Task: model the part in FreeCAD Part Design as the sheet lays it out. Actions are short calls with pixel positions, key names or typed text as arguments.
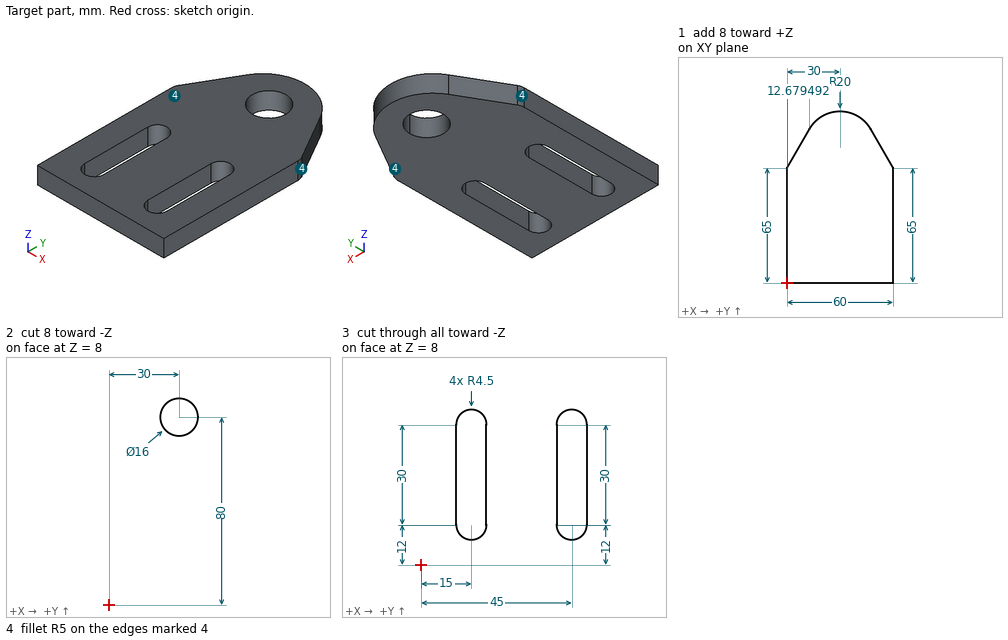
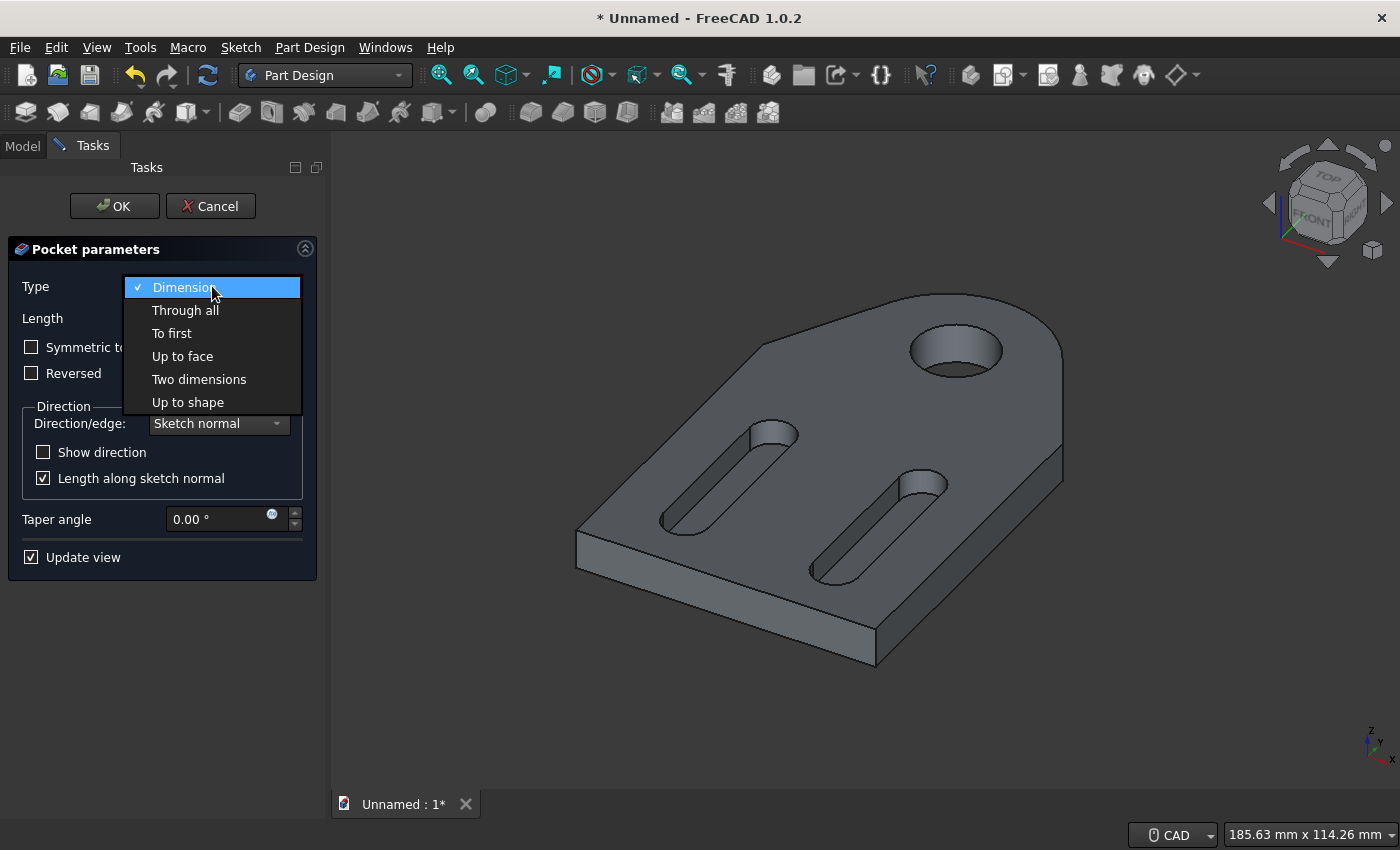
click(212, 310)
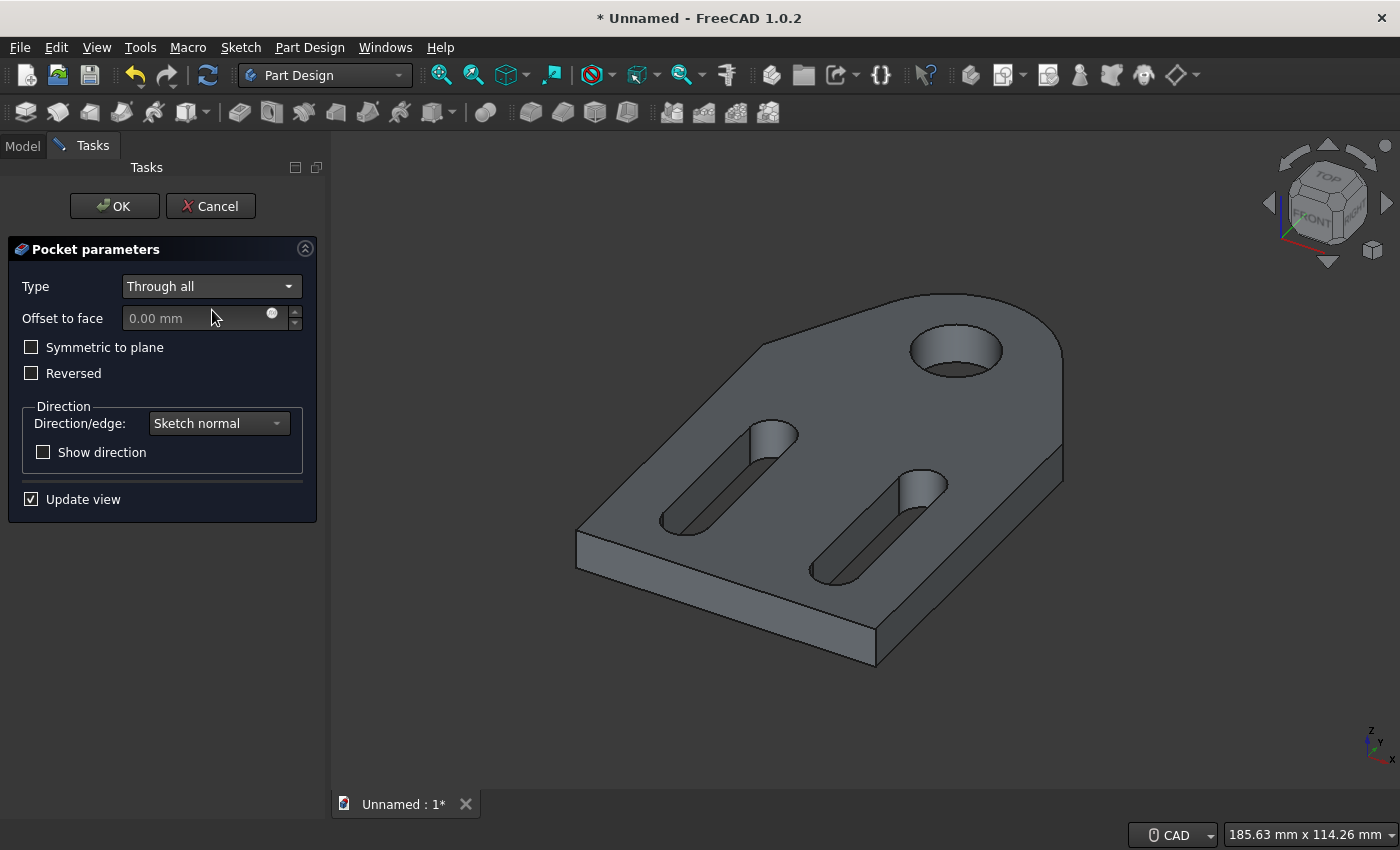
click(115, 206)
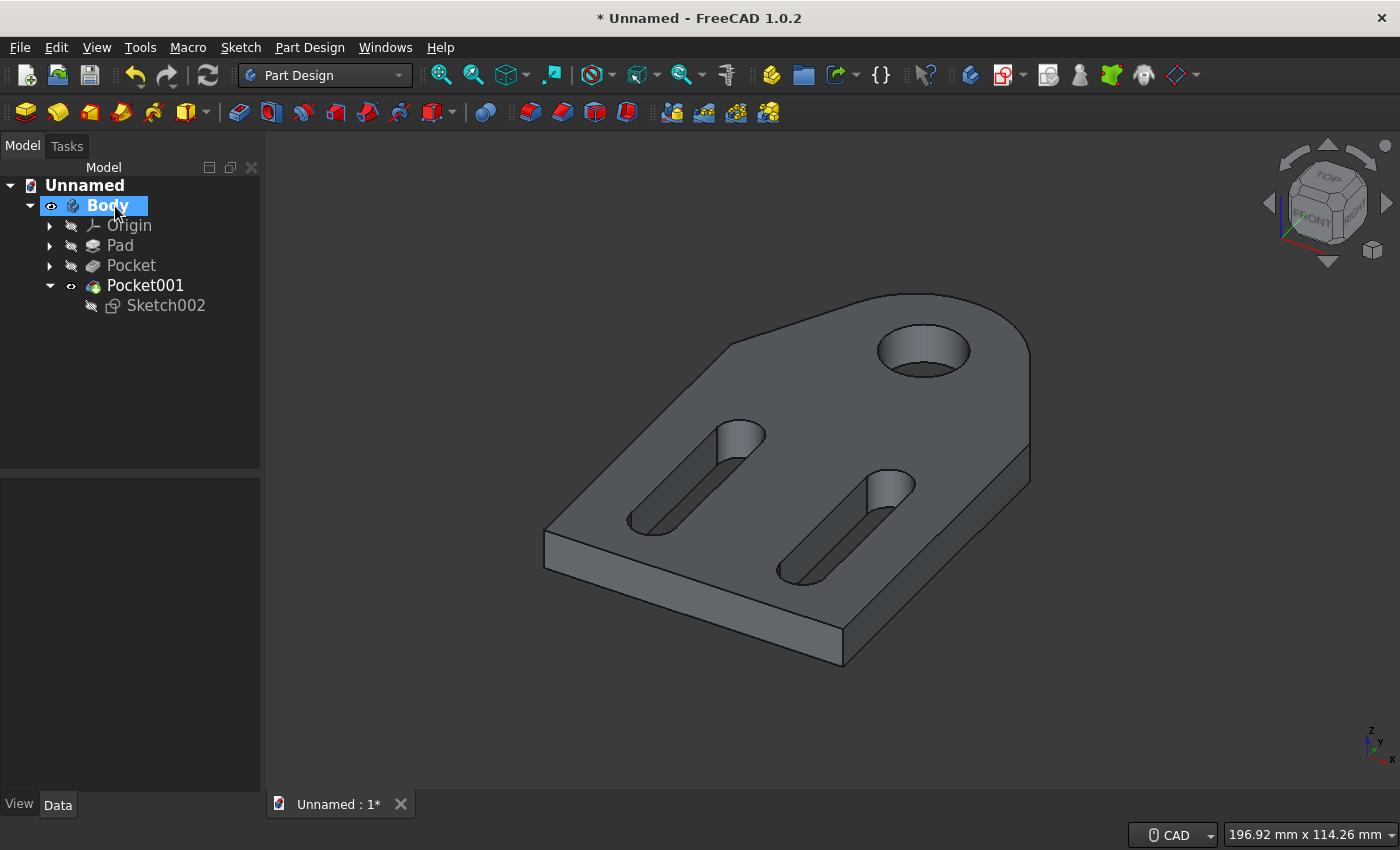
key(0)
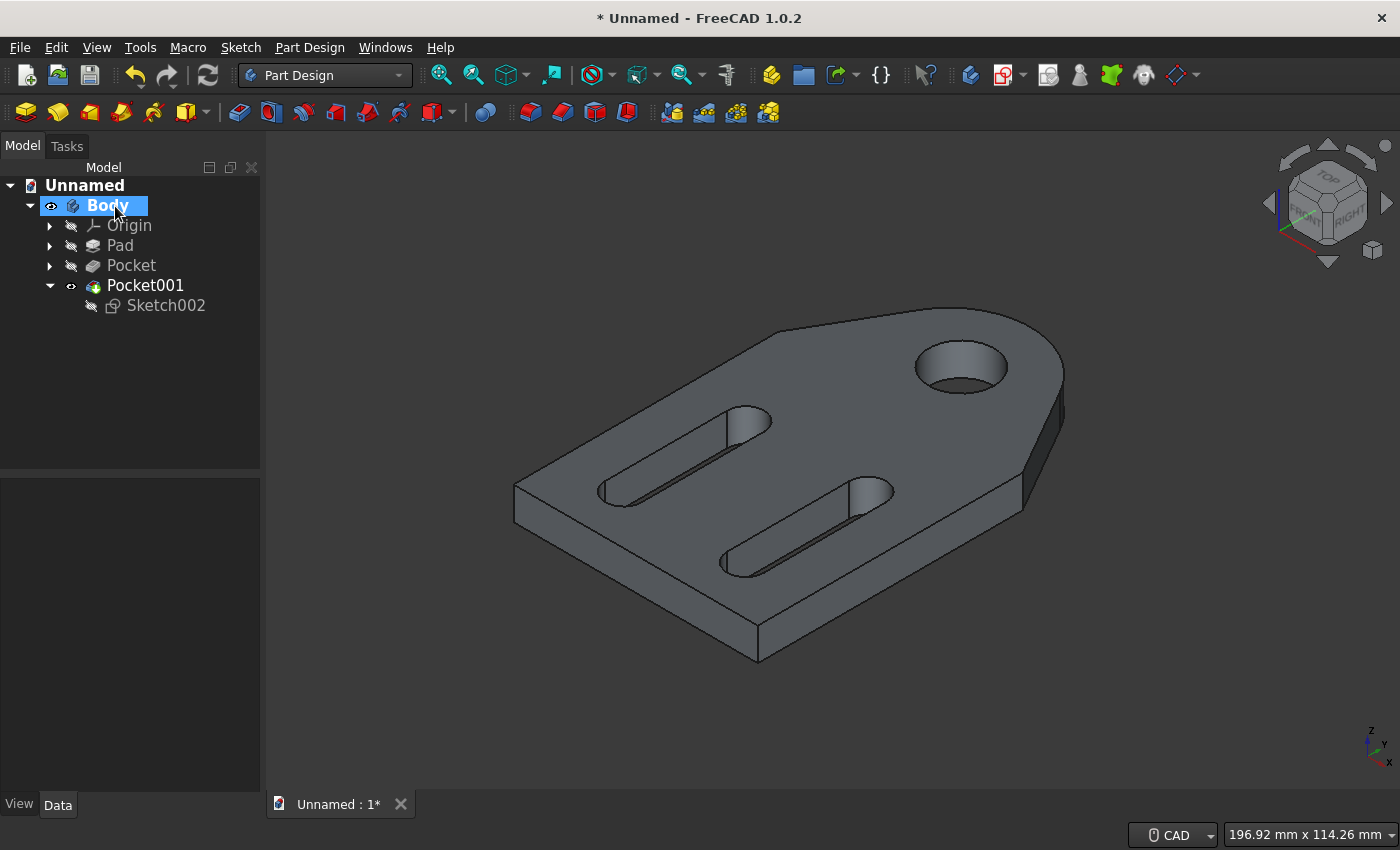
key(2)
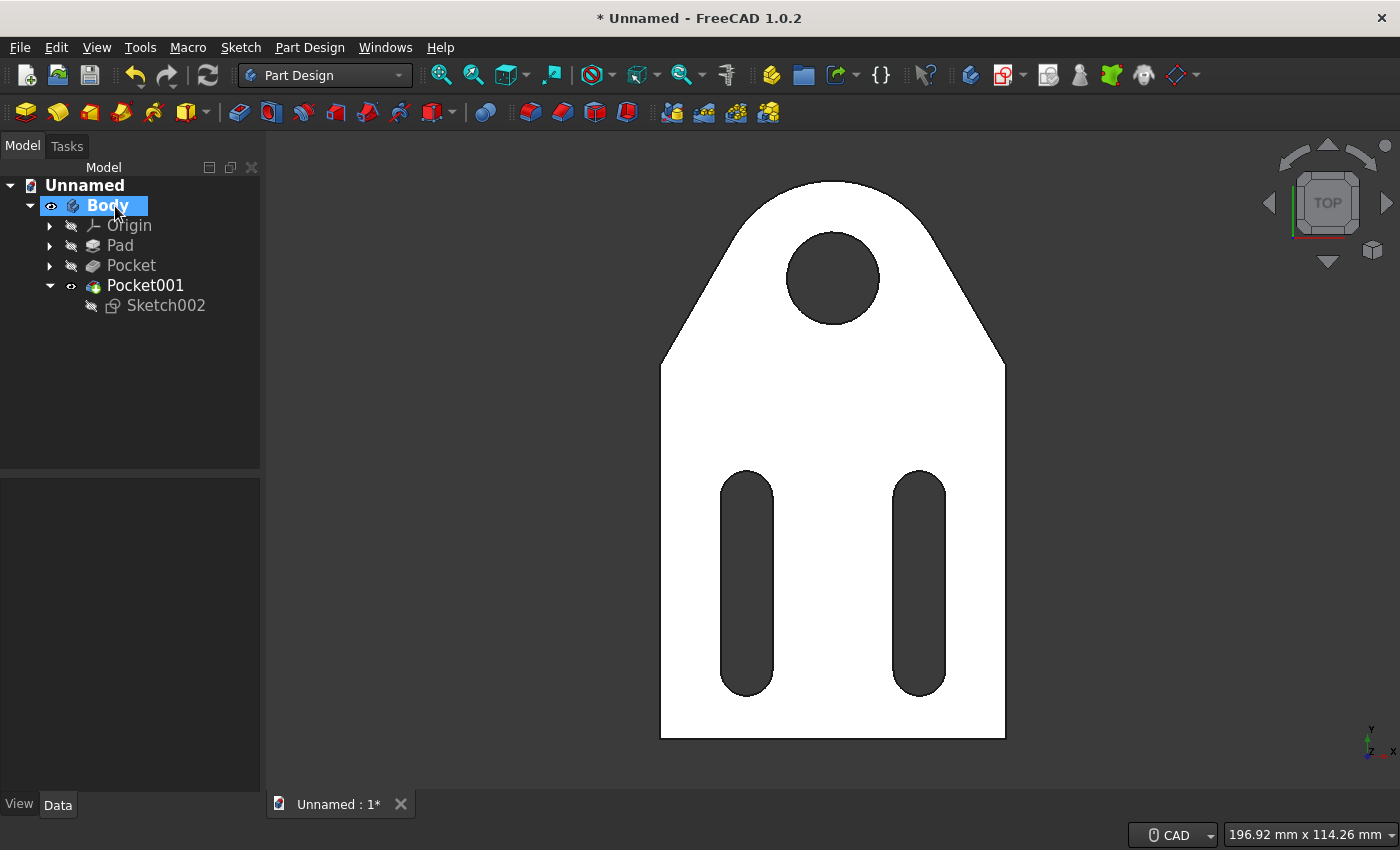
key(1)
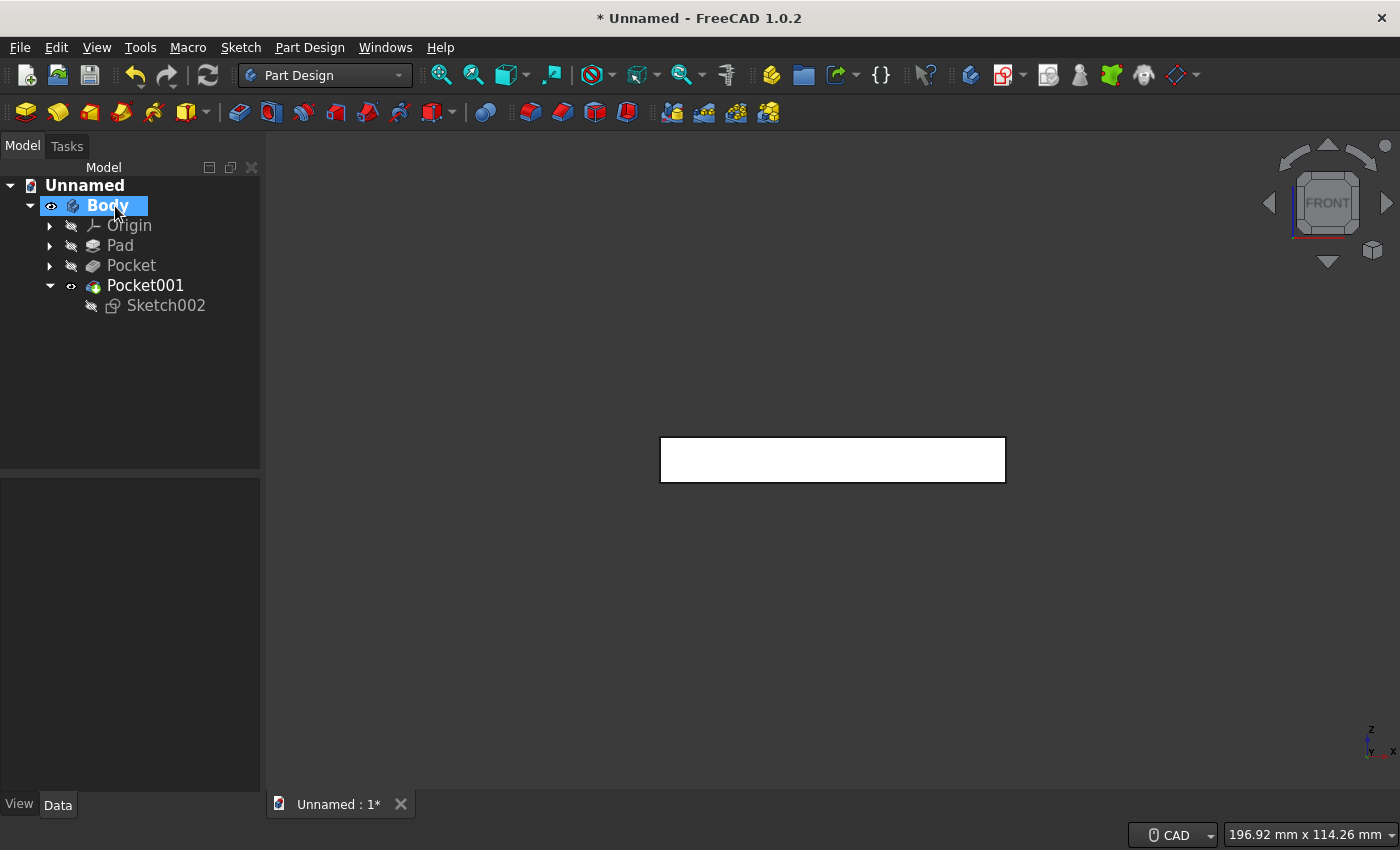
key(v)
key(f)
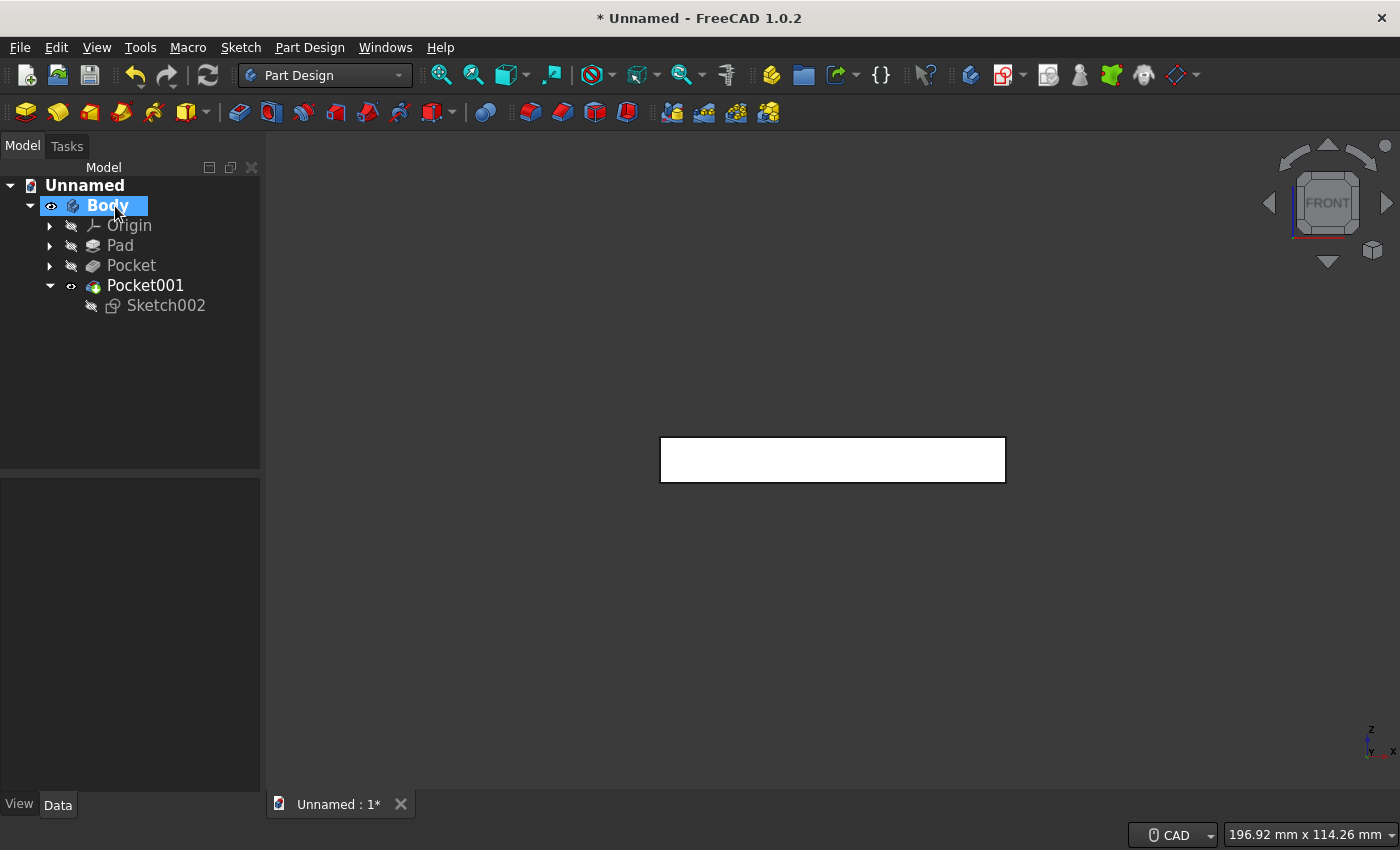
key(3)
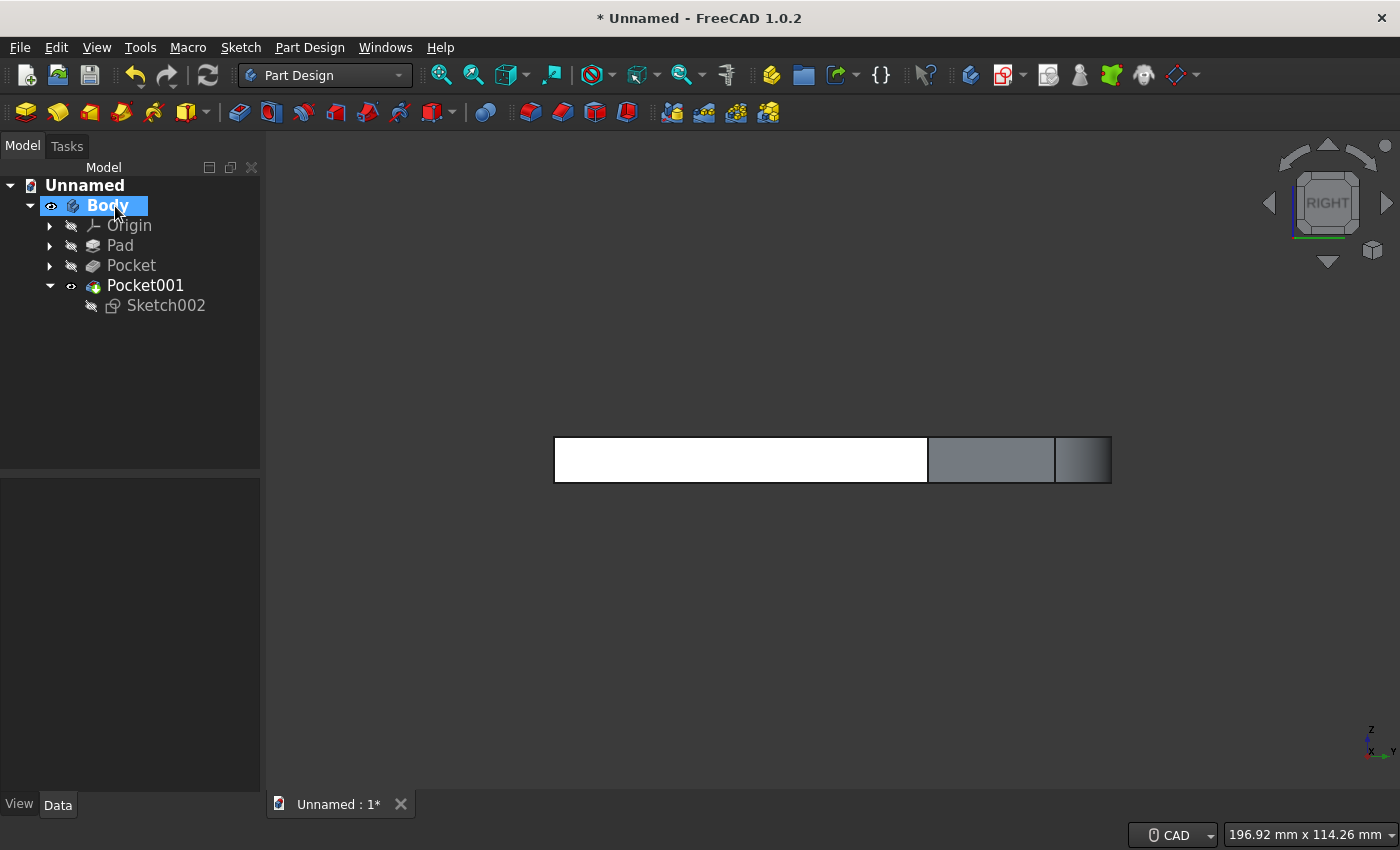
click(928, 459)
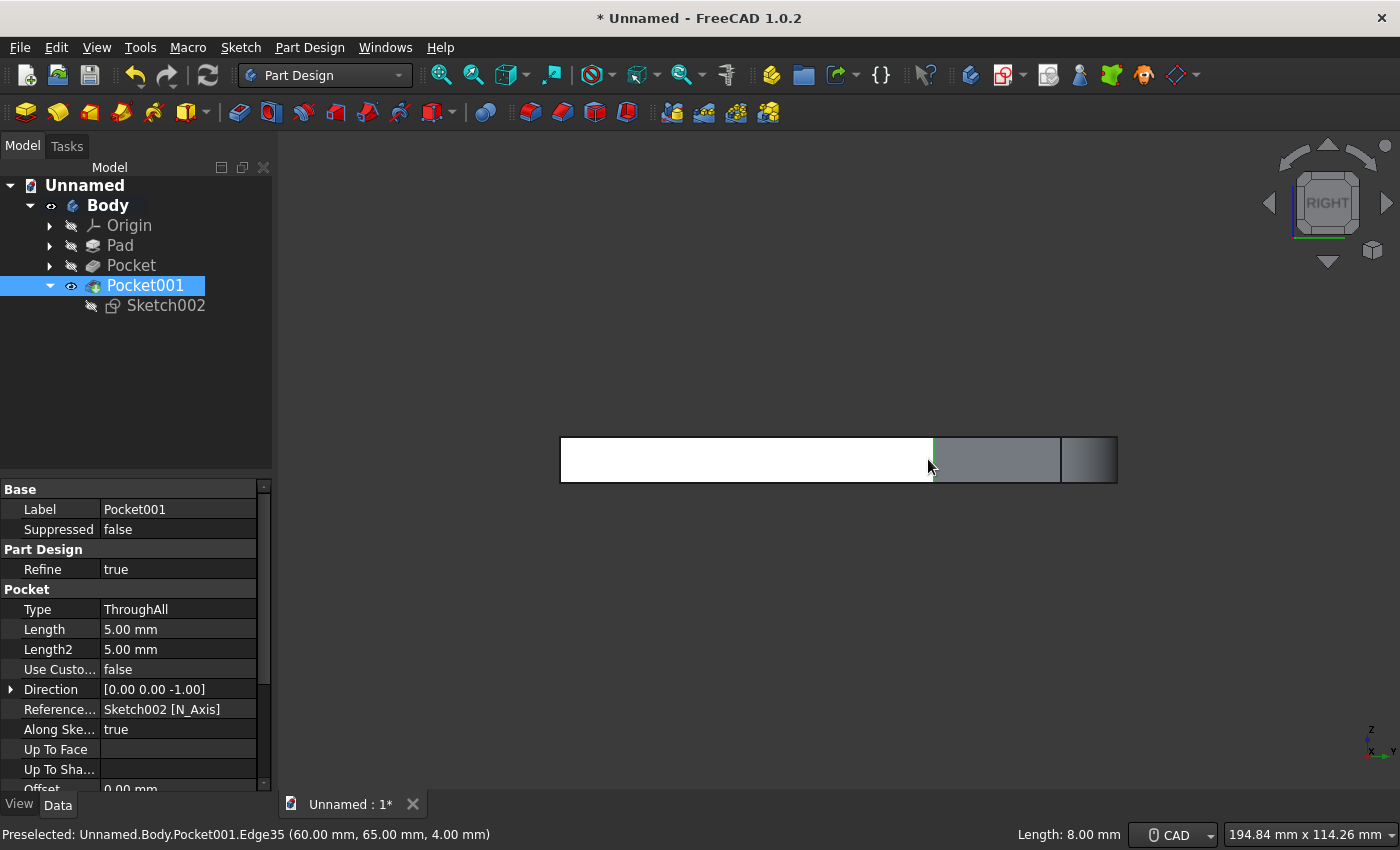
key(5)